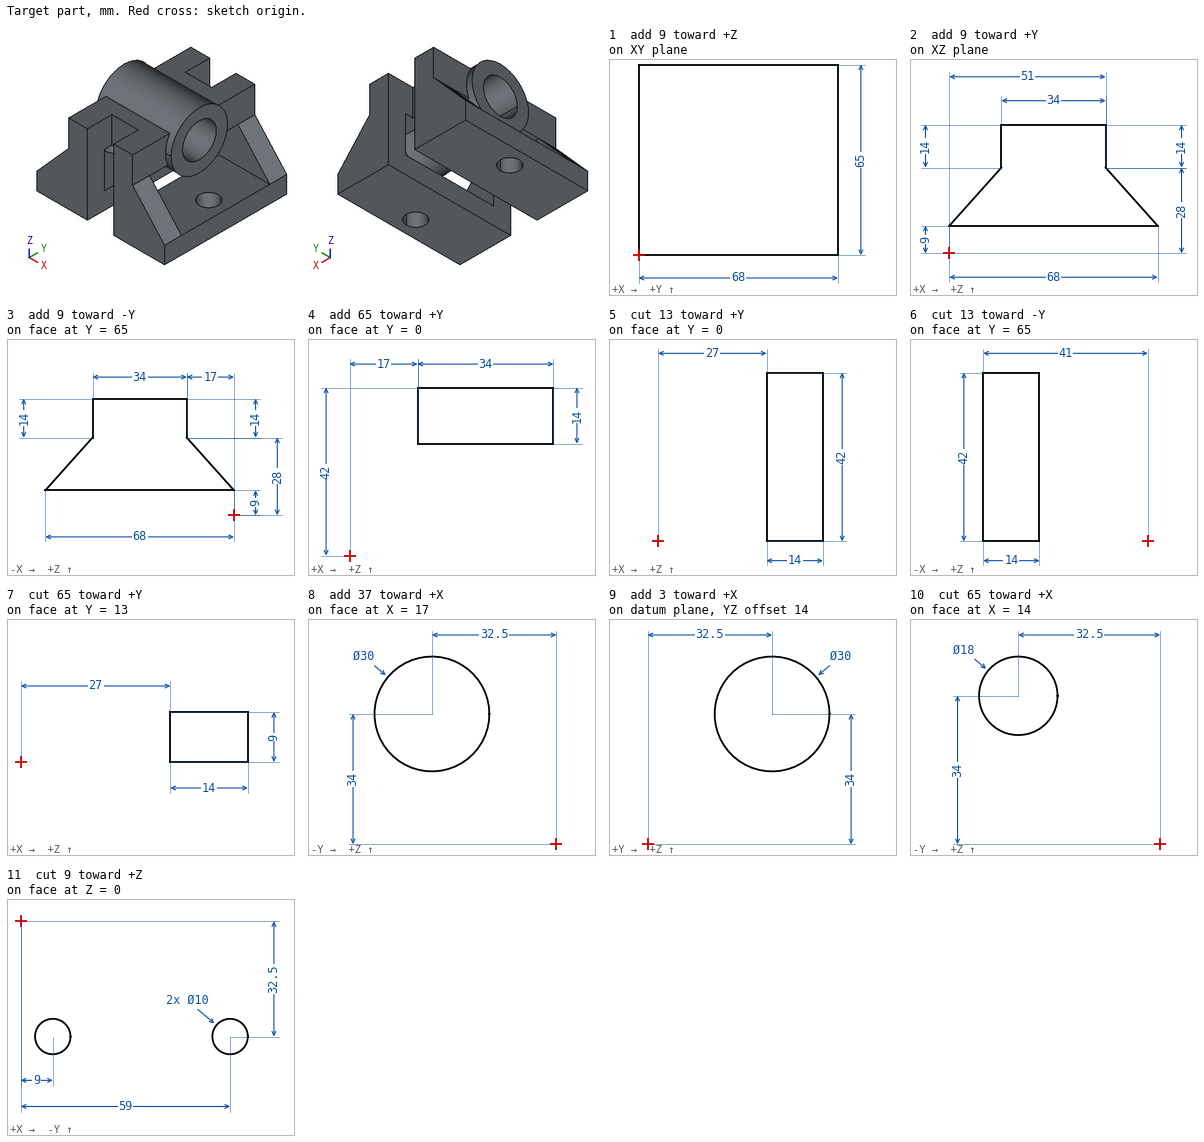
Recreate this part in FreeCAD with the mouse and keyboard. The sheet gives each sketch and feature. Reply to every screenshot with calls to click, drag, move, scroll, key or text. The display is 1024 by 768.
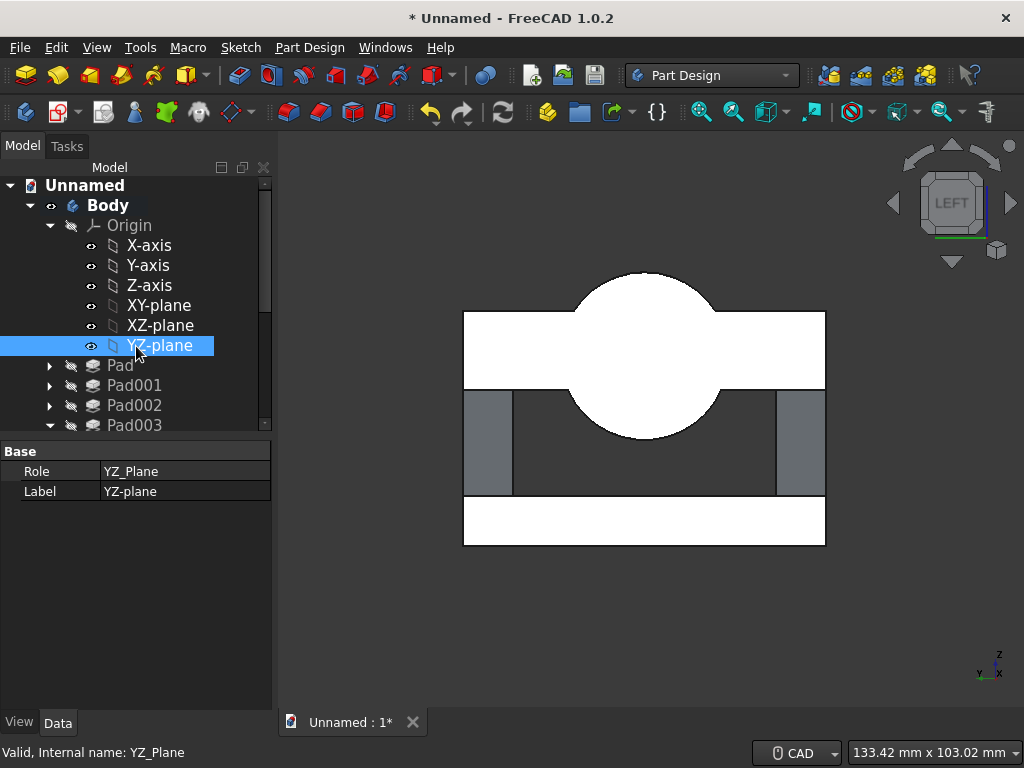
click(232, 112)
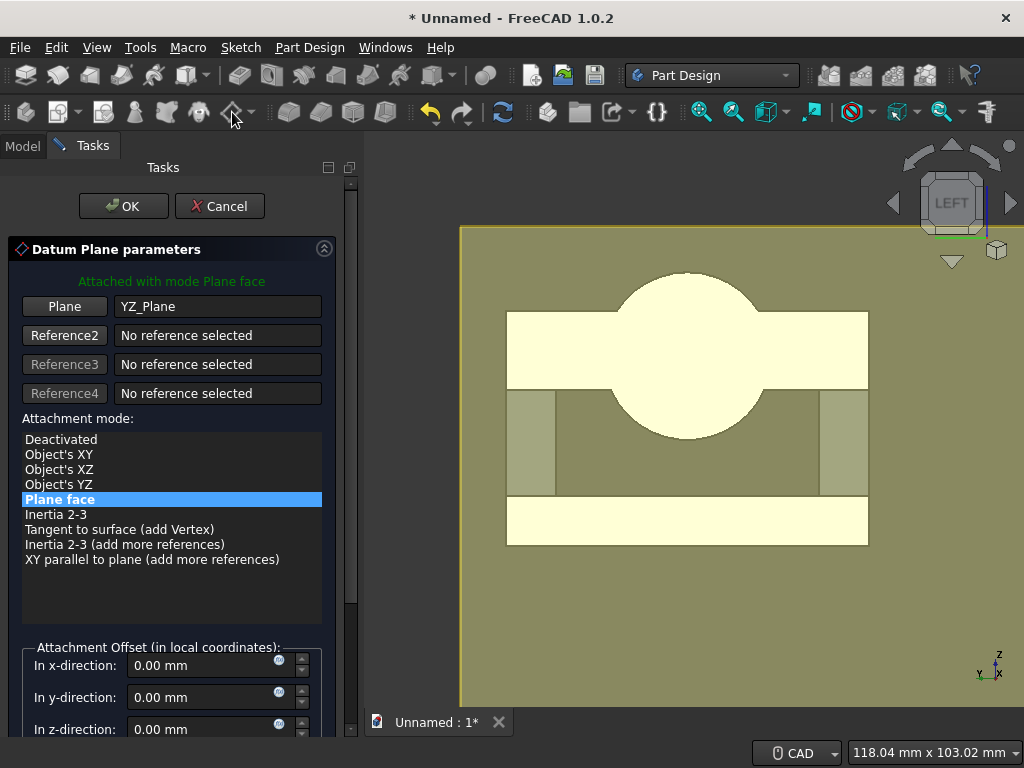
scroll(351, 456, down, 2)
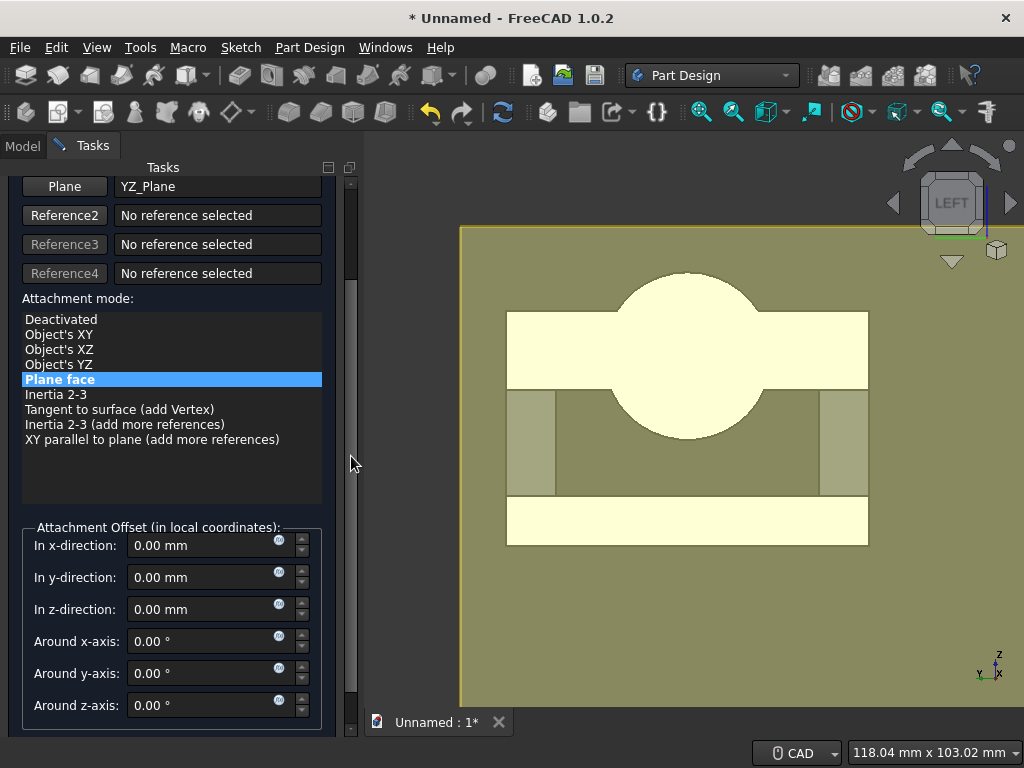
triple_click(210, 609)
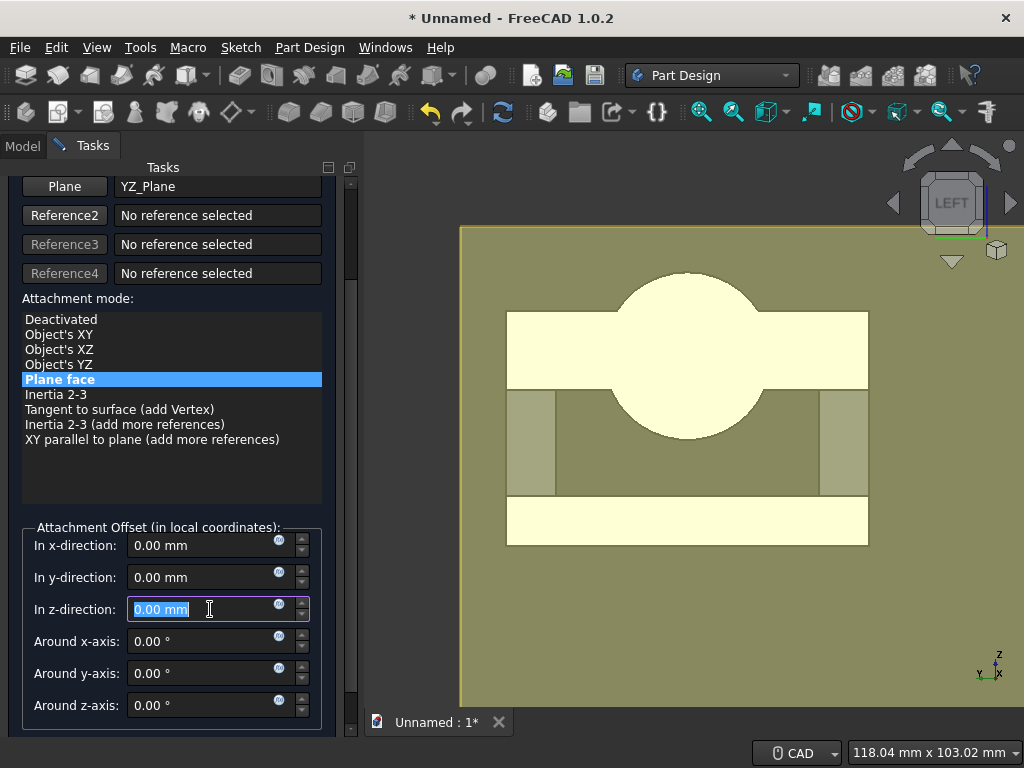
text(14)
key(Tab)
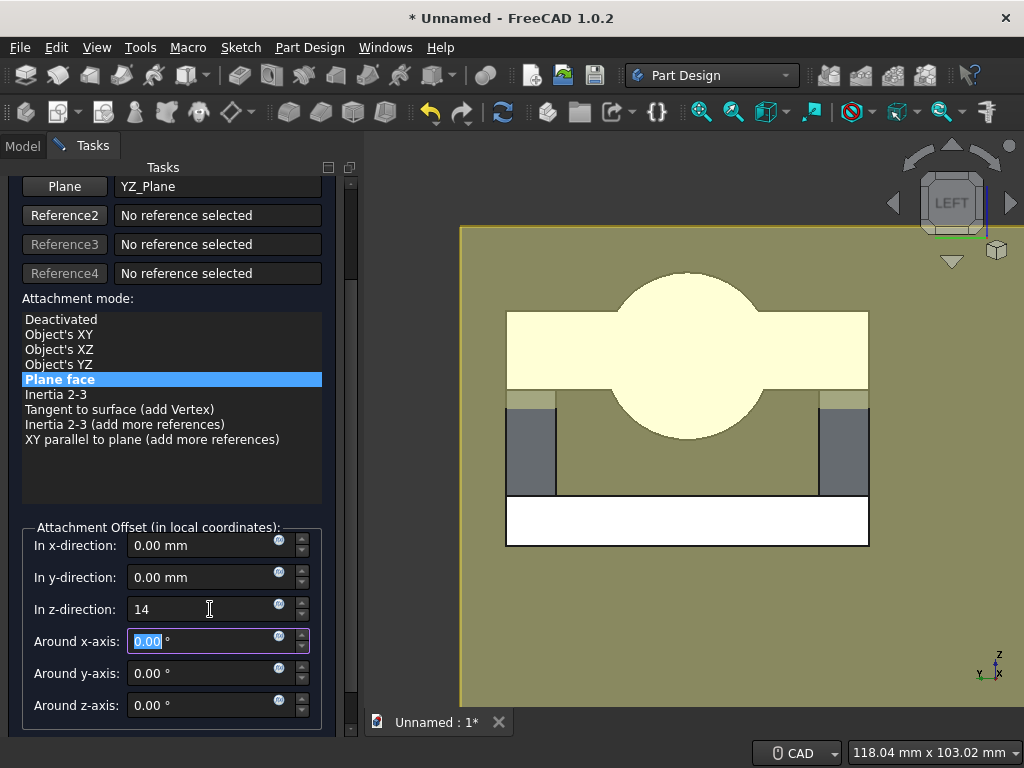
scroll(351, 456, up, 3)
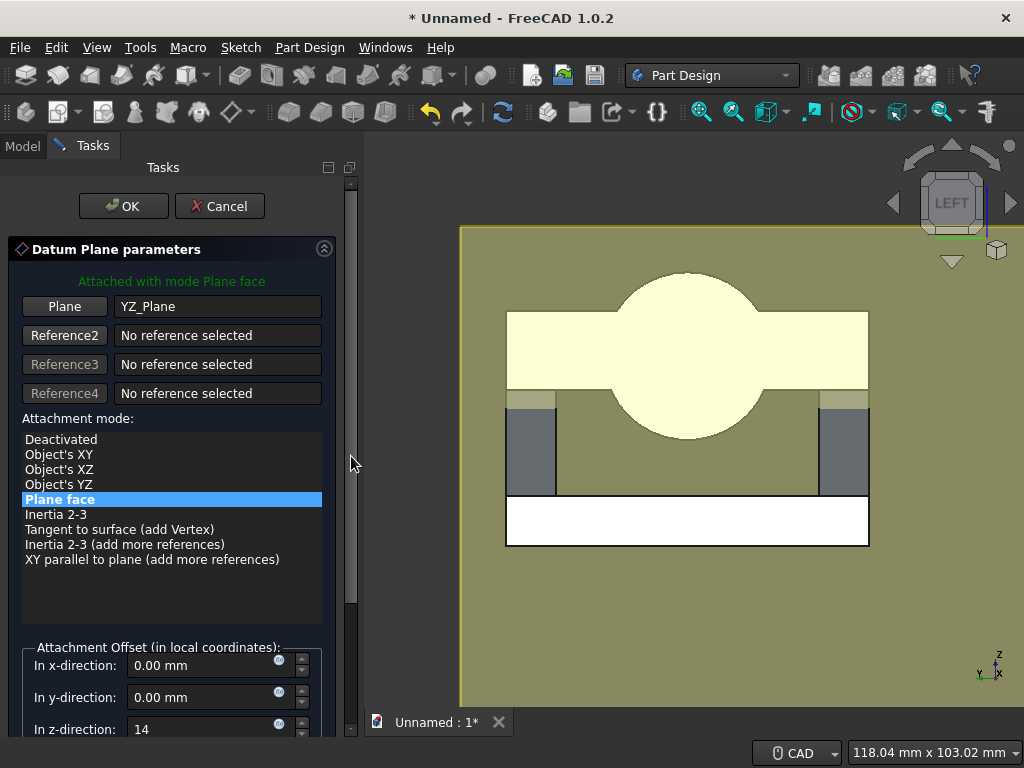
click(124, 206)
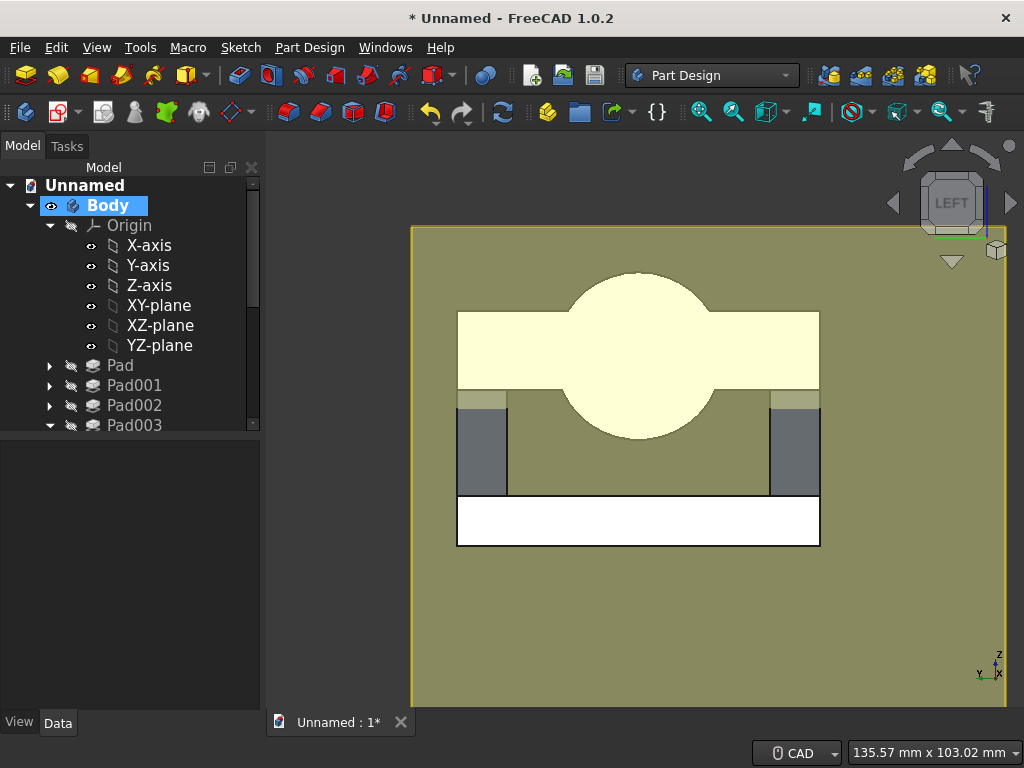
scroll(100, 301, down, 3)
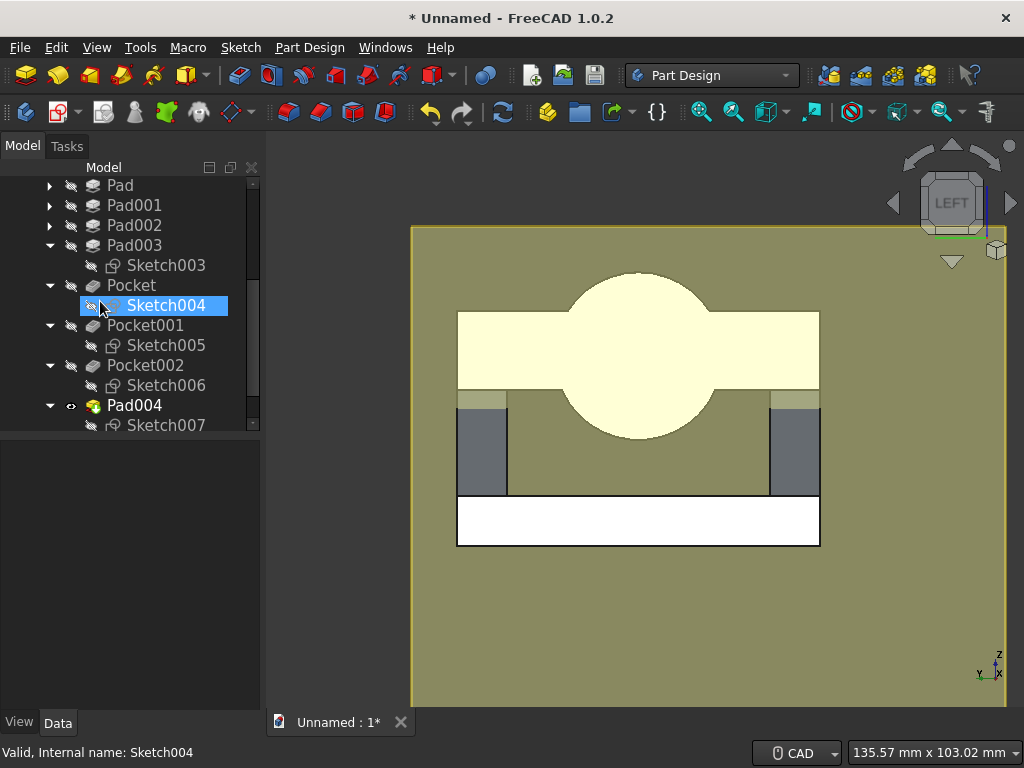
scroll(140, 301, up, 15)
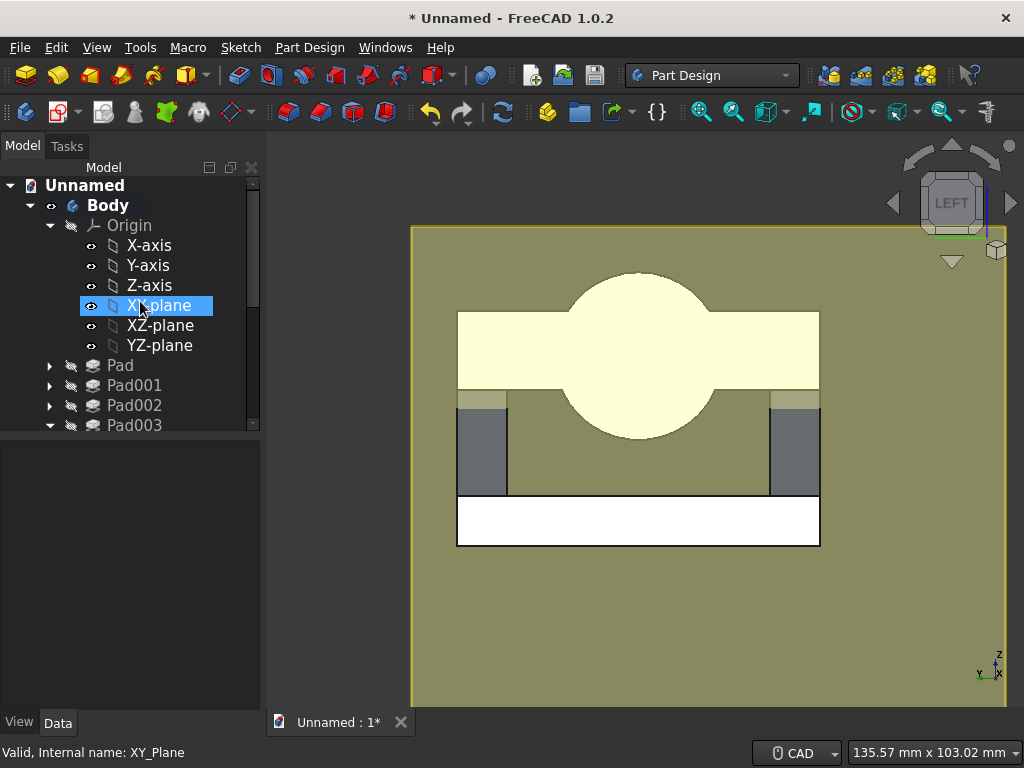
scroll(100, 301, down, 6)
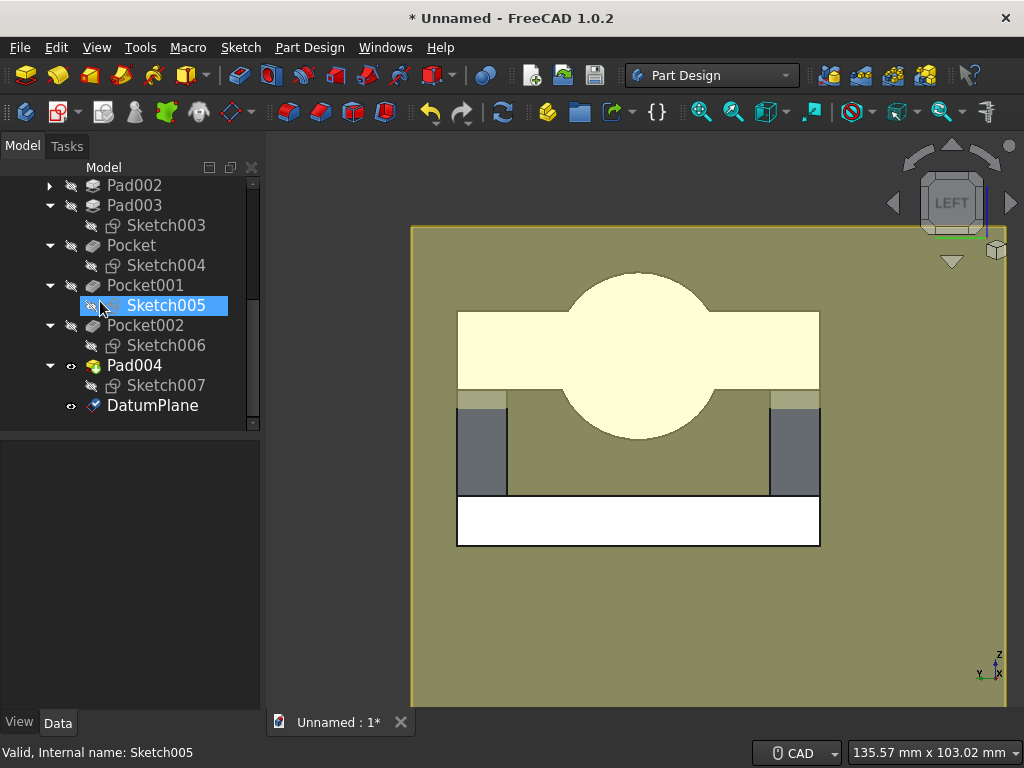
click(116, 406)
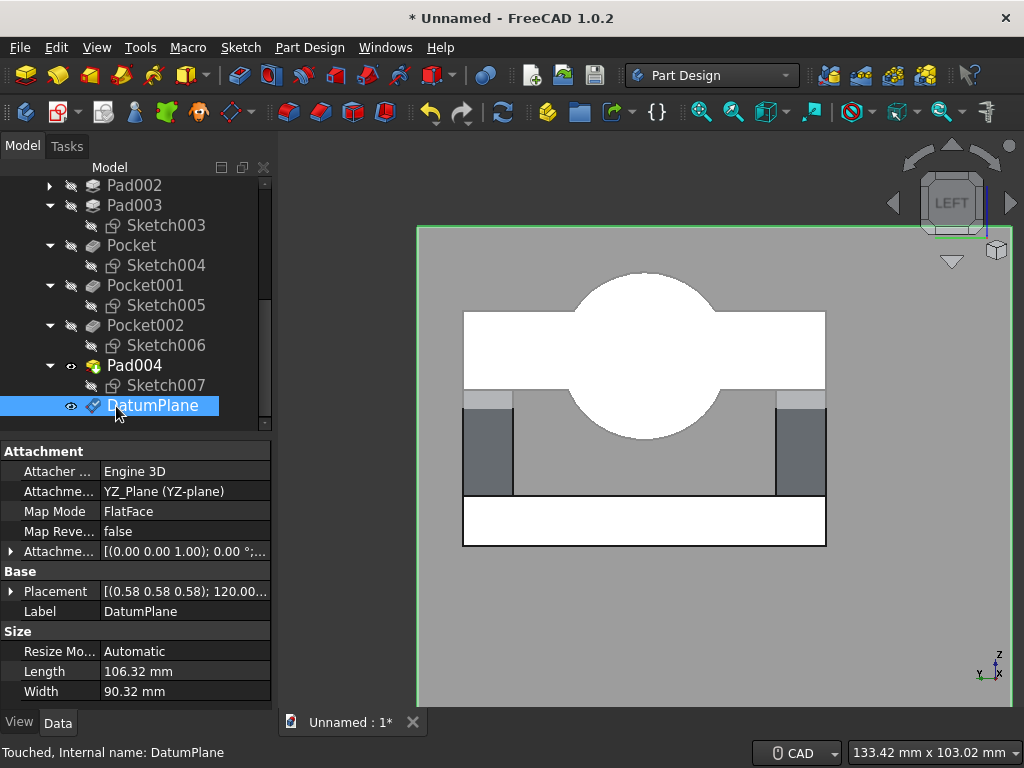
click(58, 112)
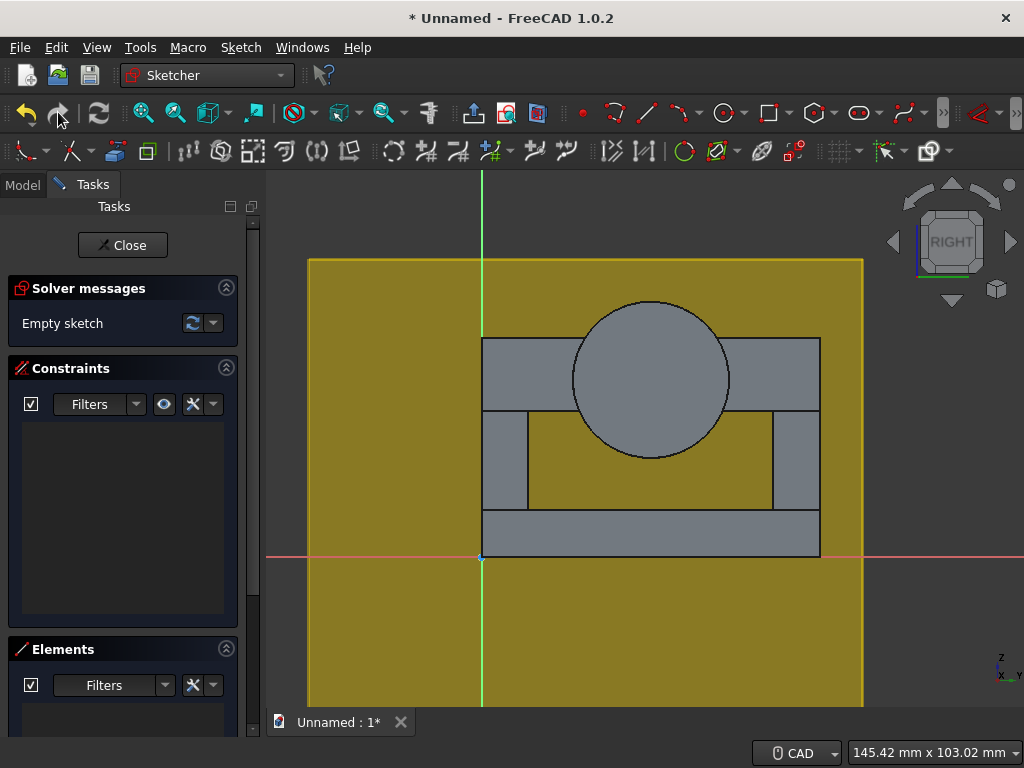
click(538, 114)